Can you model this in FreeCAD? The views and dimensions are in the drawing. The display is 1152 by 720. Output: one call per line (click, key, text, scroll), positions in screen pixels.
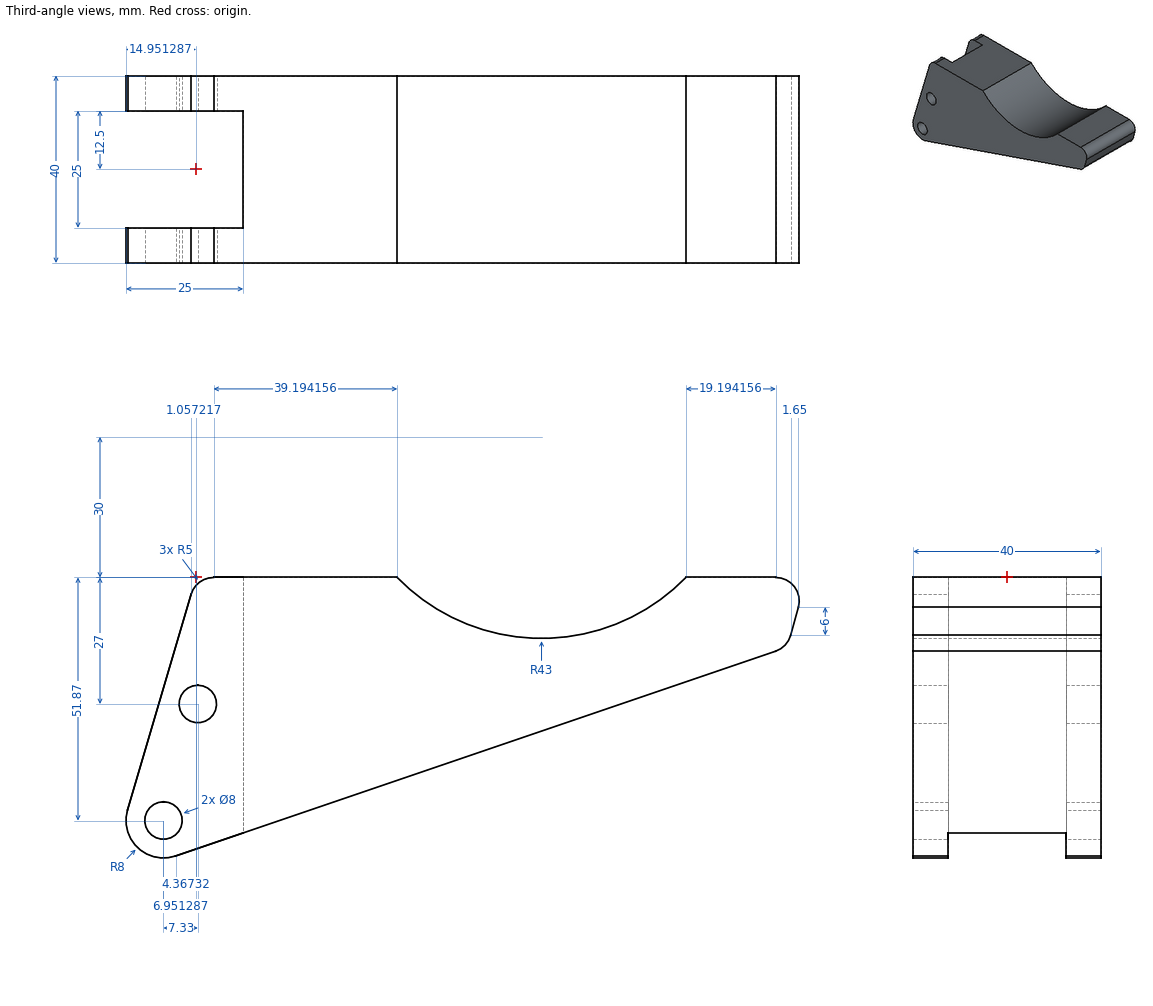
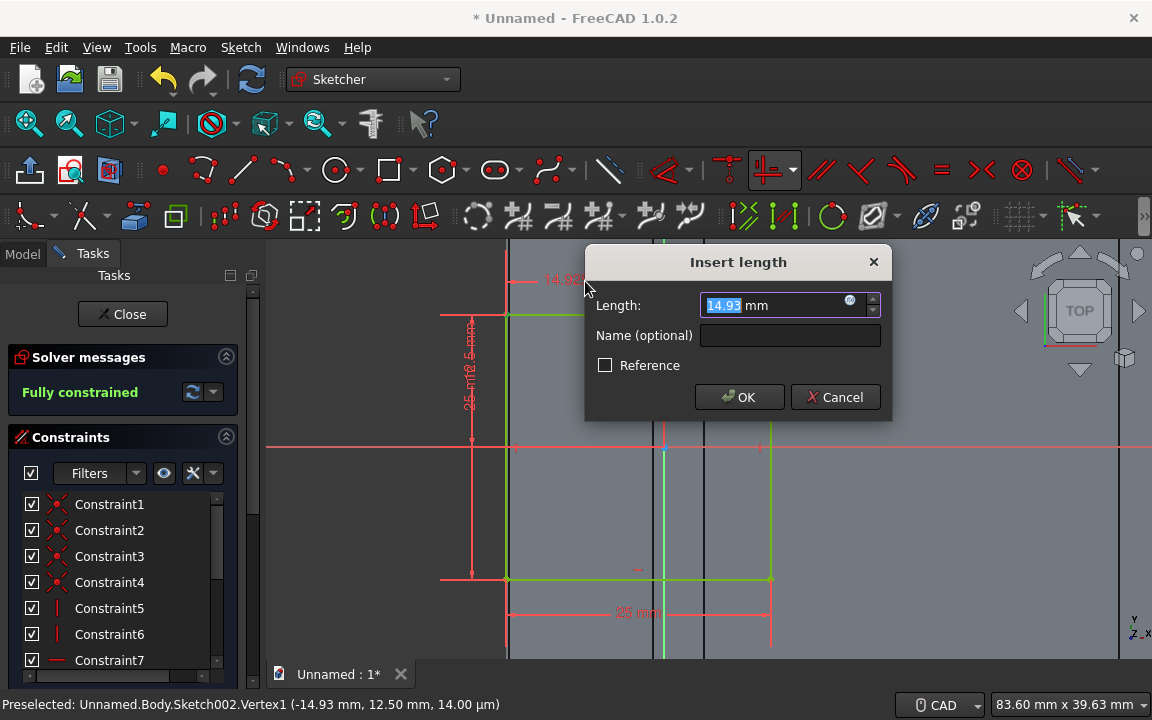
text(14.951287)
key(Return)
key(Escape)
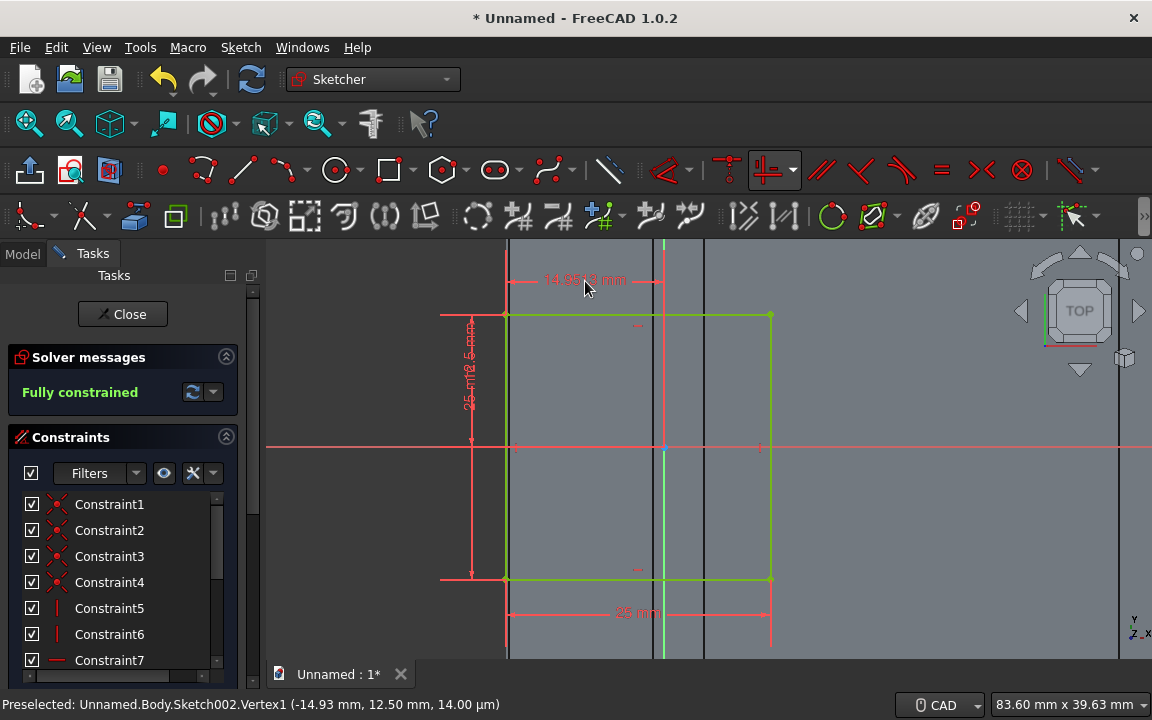
click(123, 314)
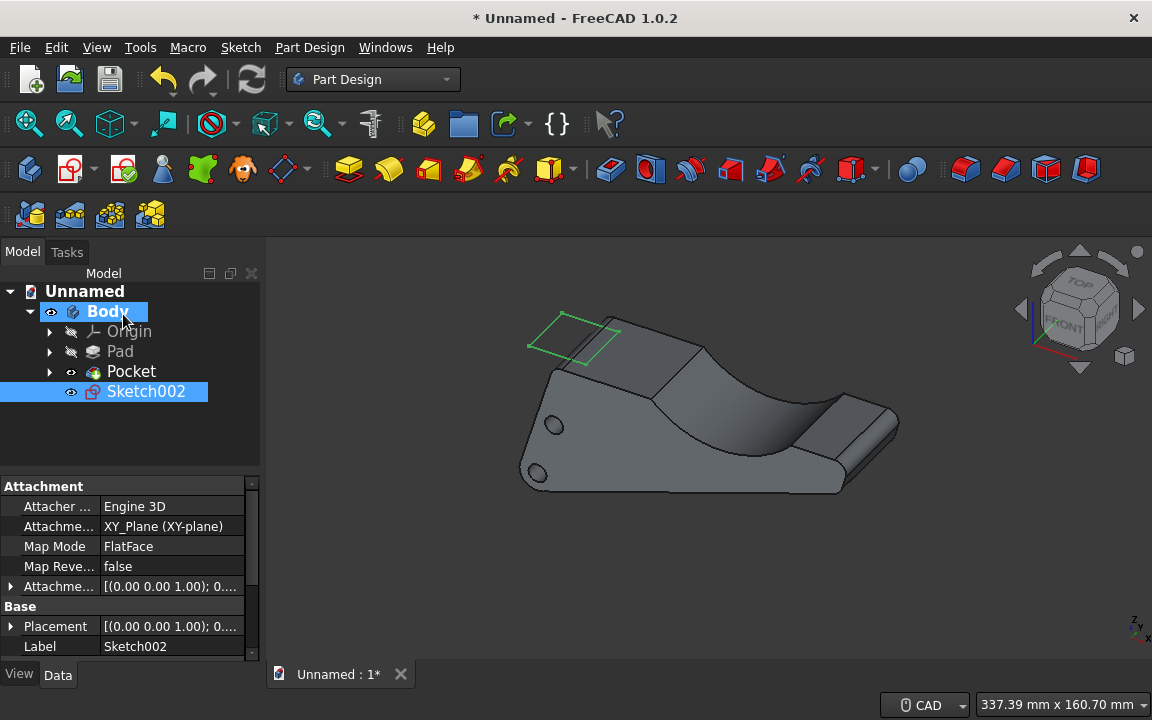
click(612, 170)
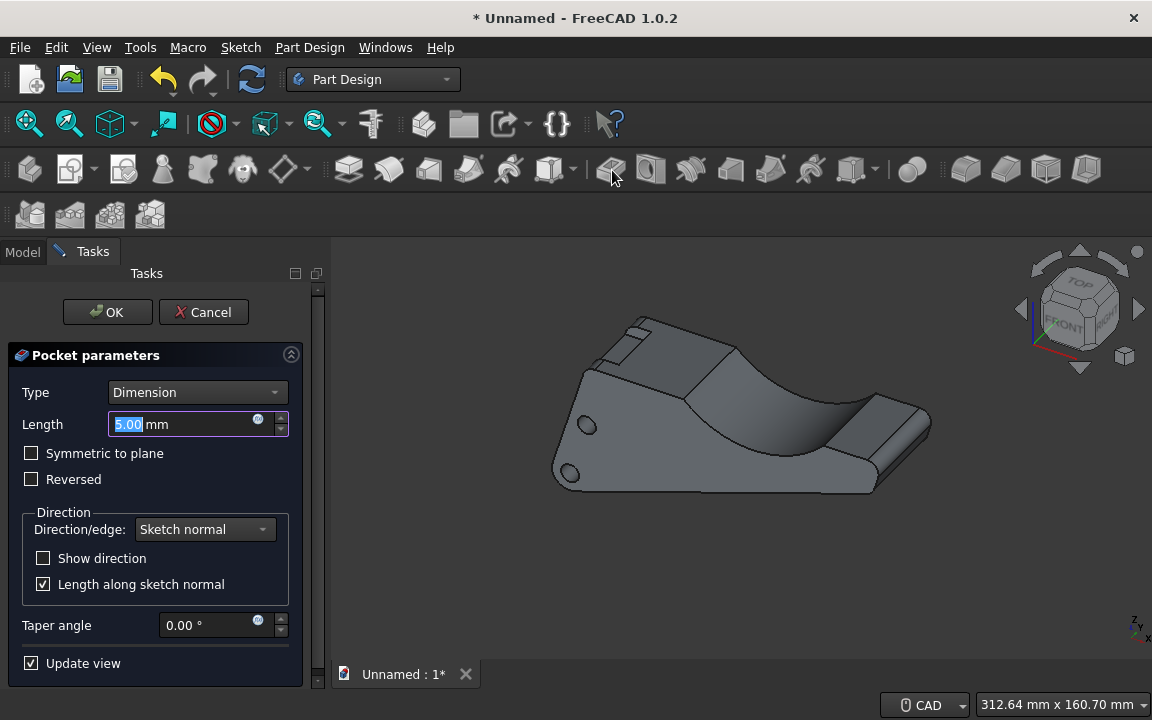
click(198, 392)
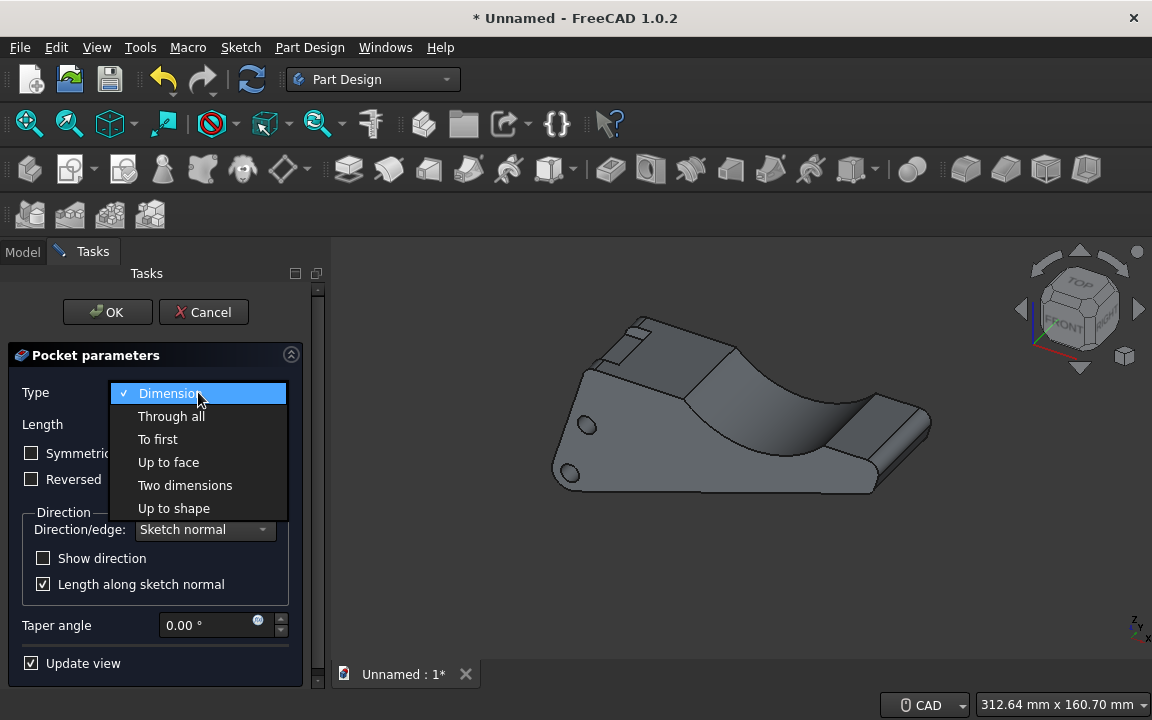
click(198, 416)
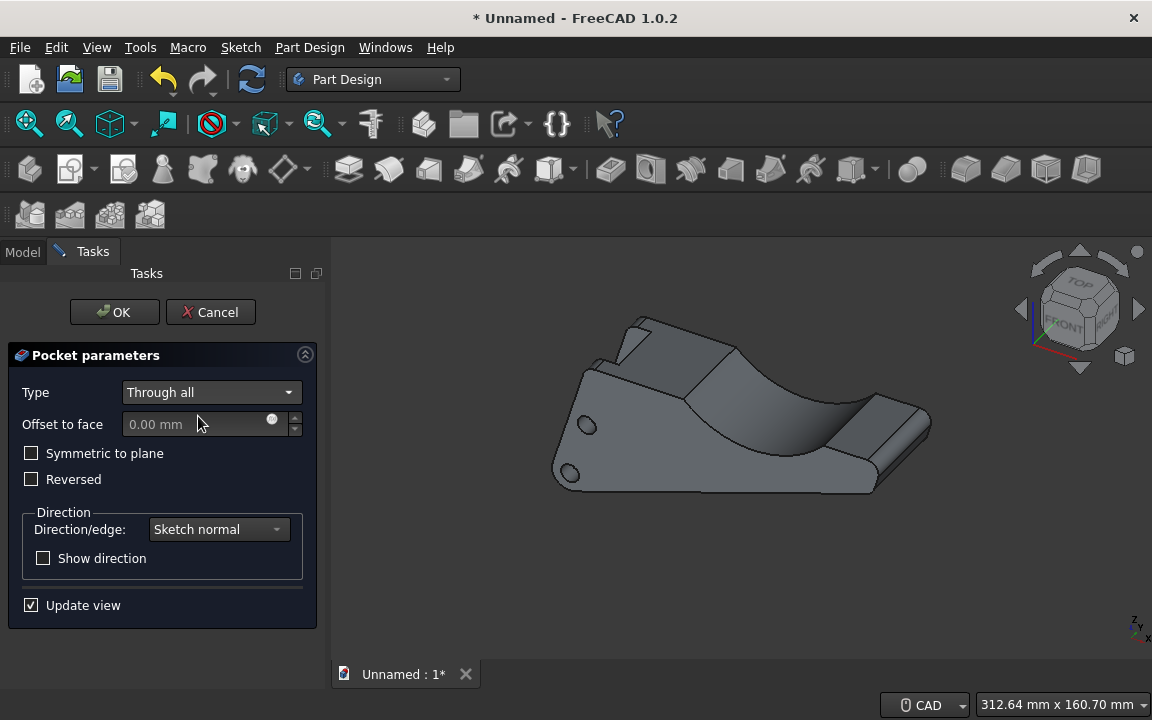
click(115, 312)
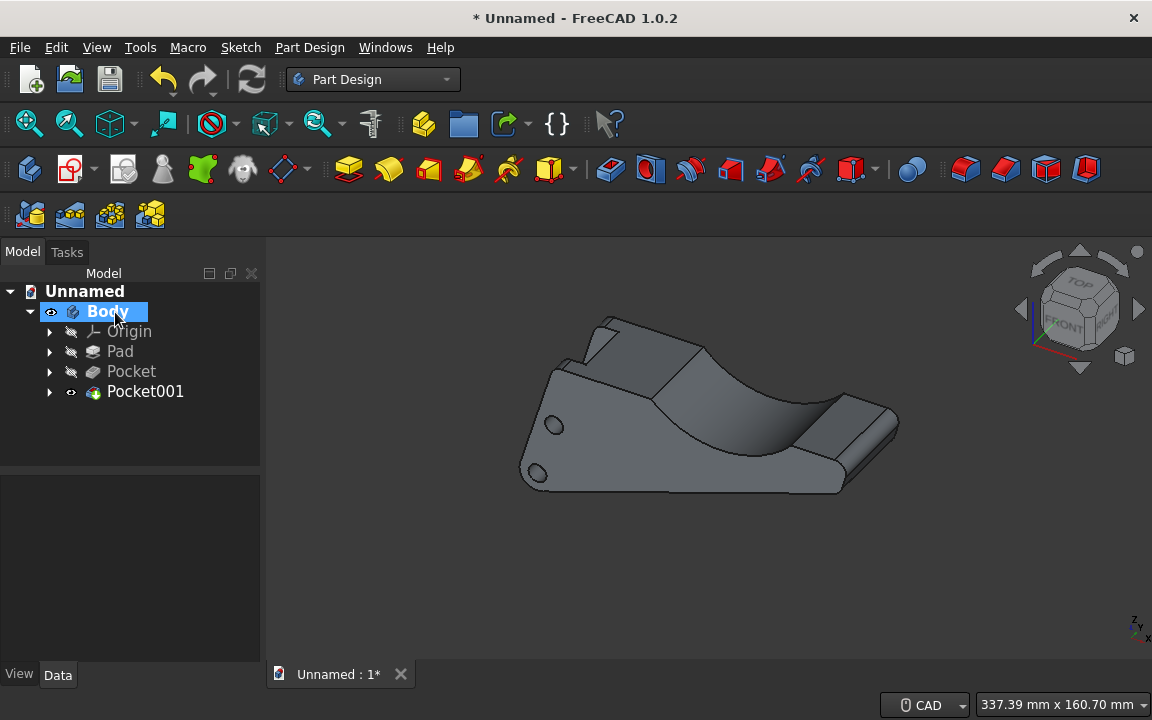
key(0)